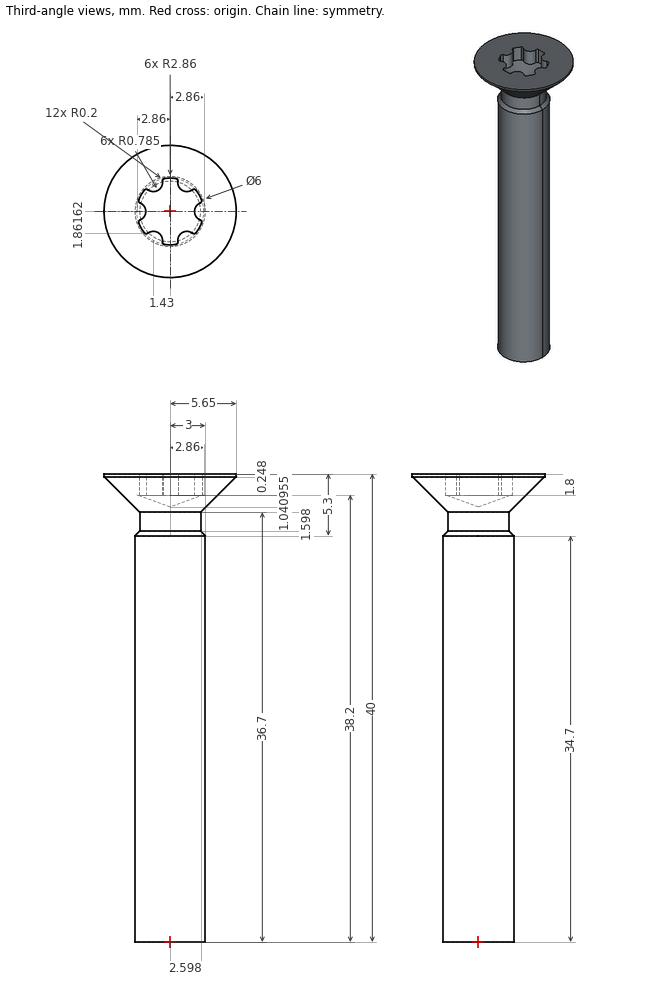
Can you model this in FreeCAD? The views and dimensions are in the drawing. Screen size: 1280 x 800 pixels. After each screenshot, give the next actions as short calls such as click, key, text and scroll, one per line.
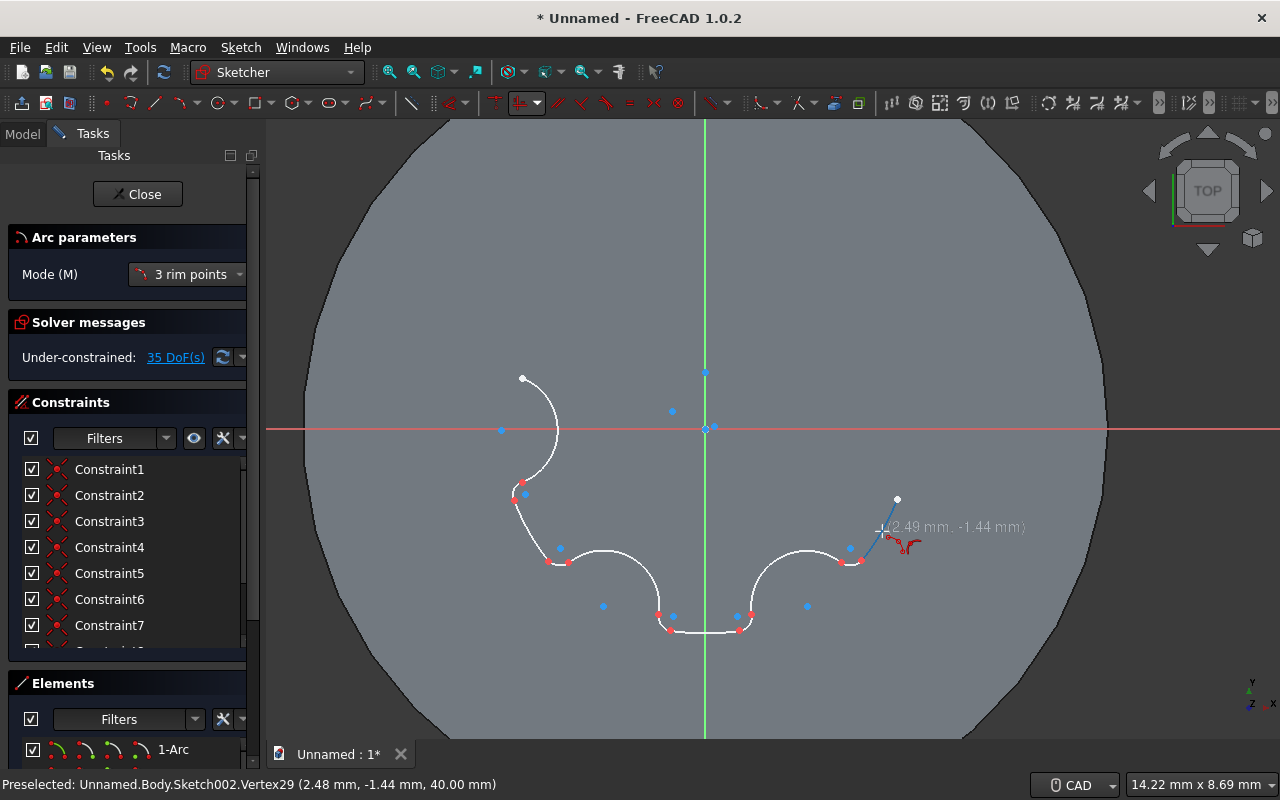
click(897, 500)
click(889, 481)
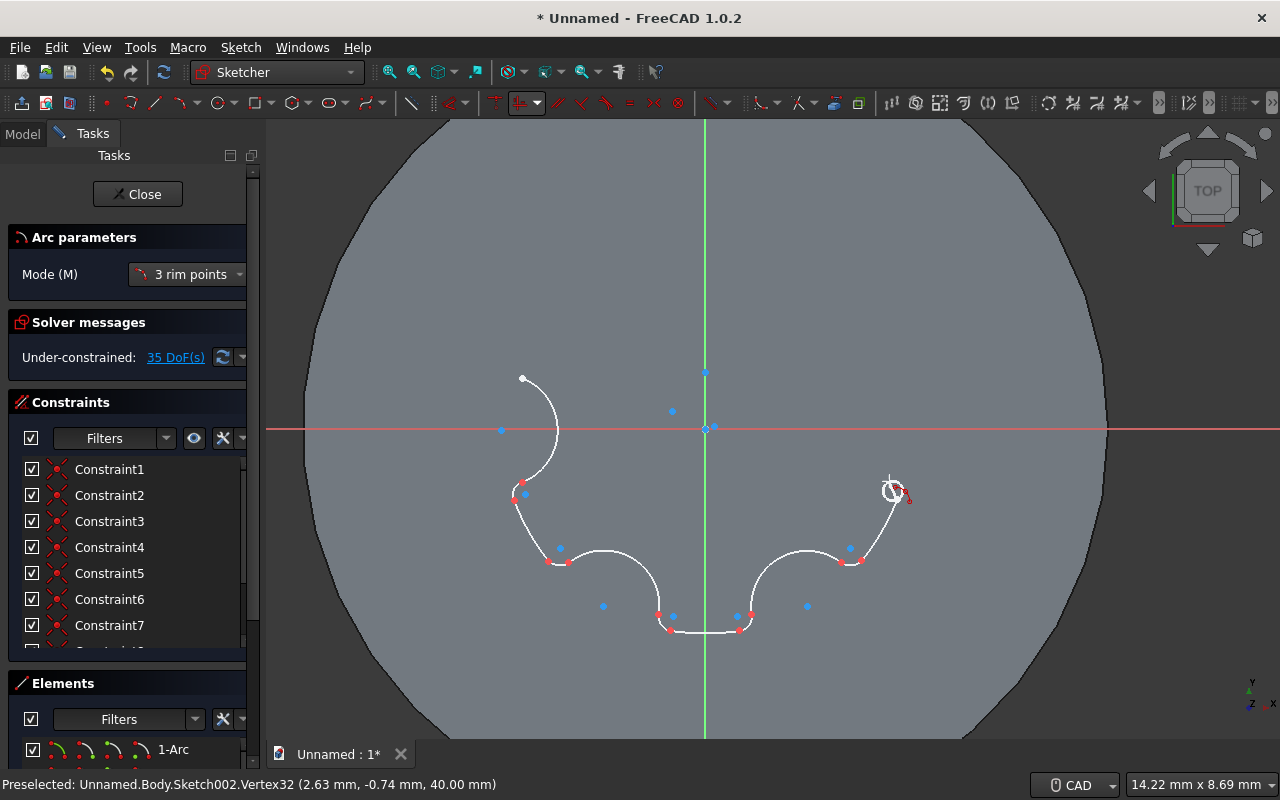
scroll(896, 489, up, 7)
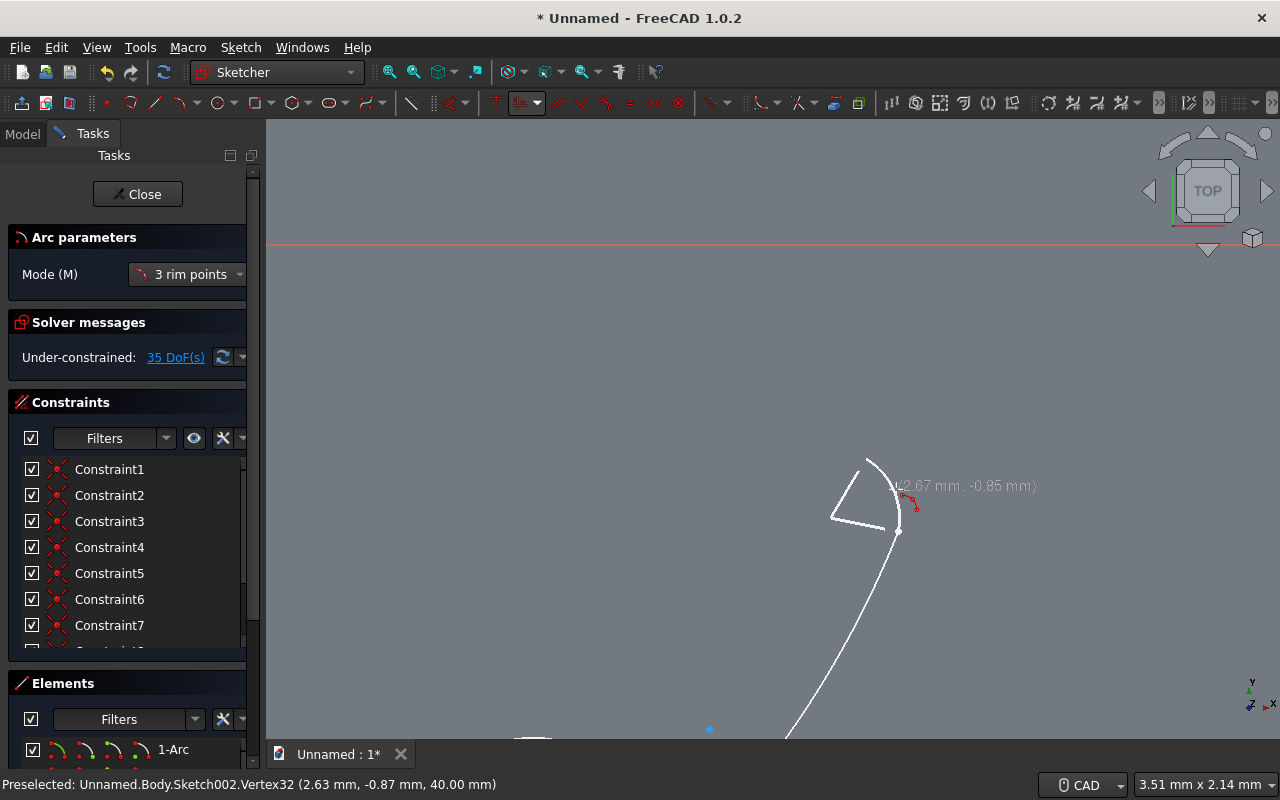
click(896, 486)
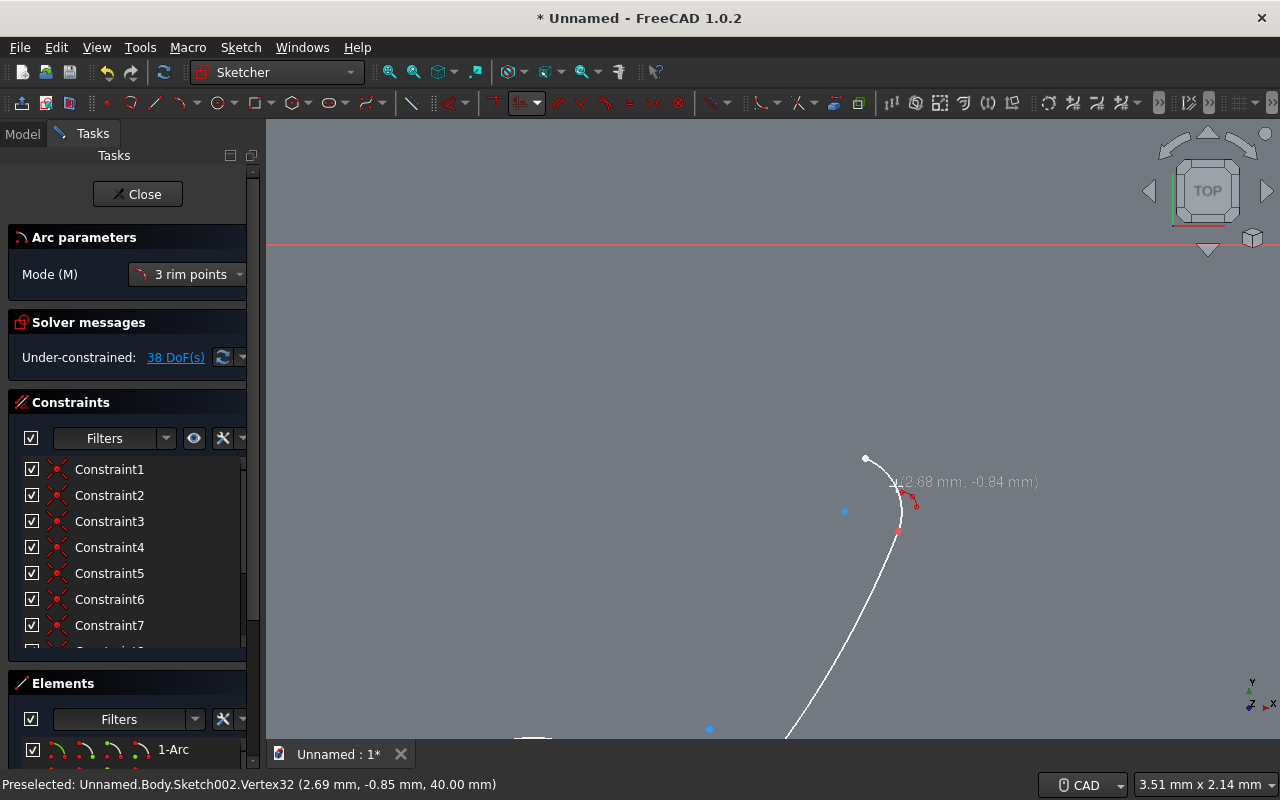
scroll(896, 489, down, 7)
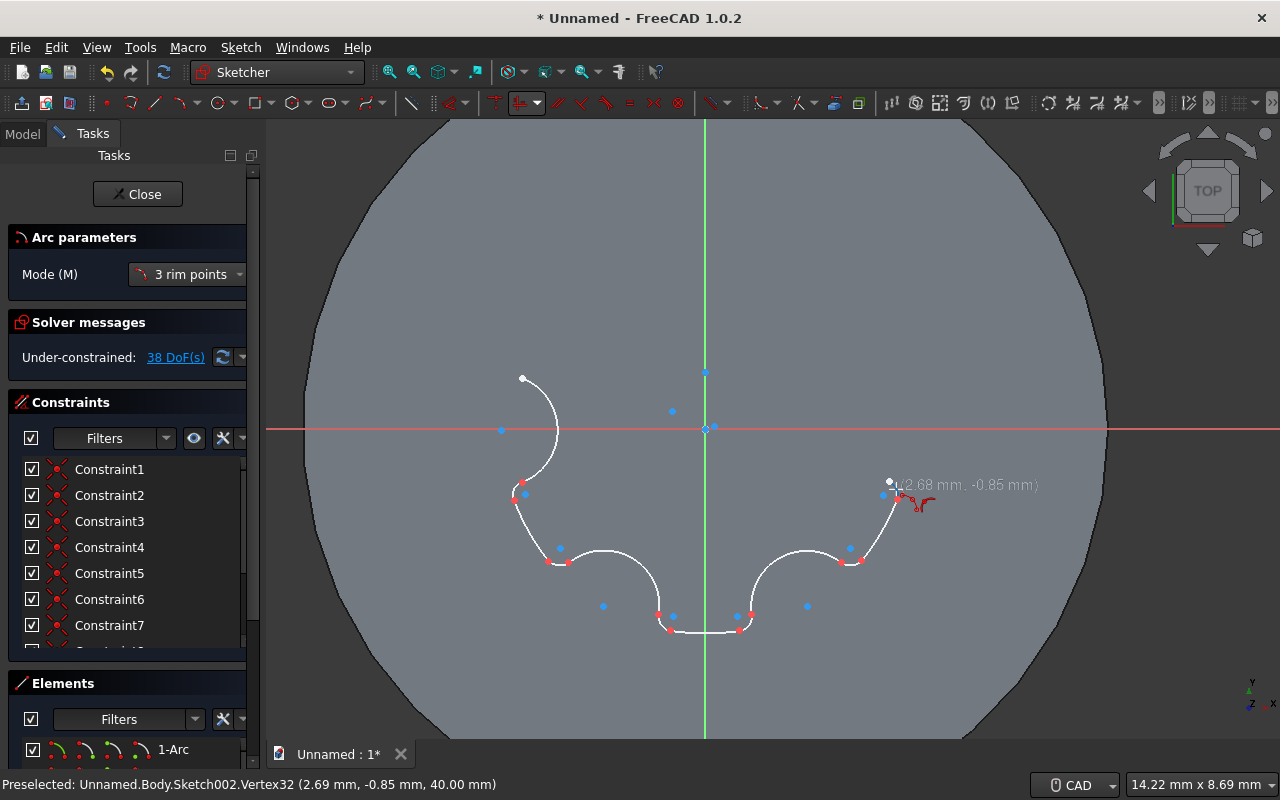
click(889, 482)
click(889, 377)
click(860, 404)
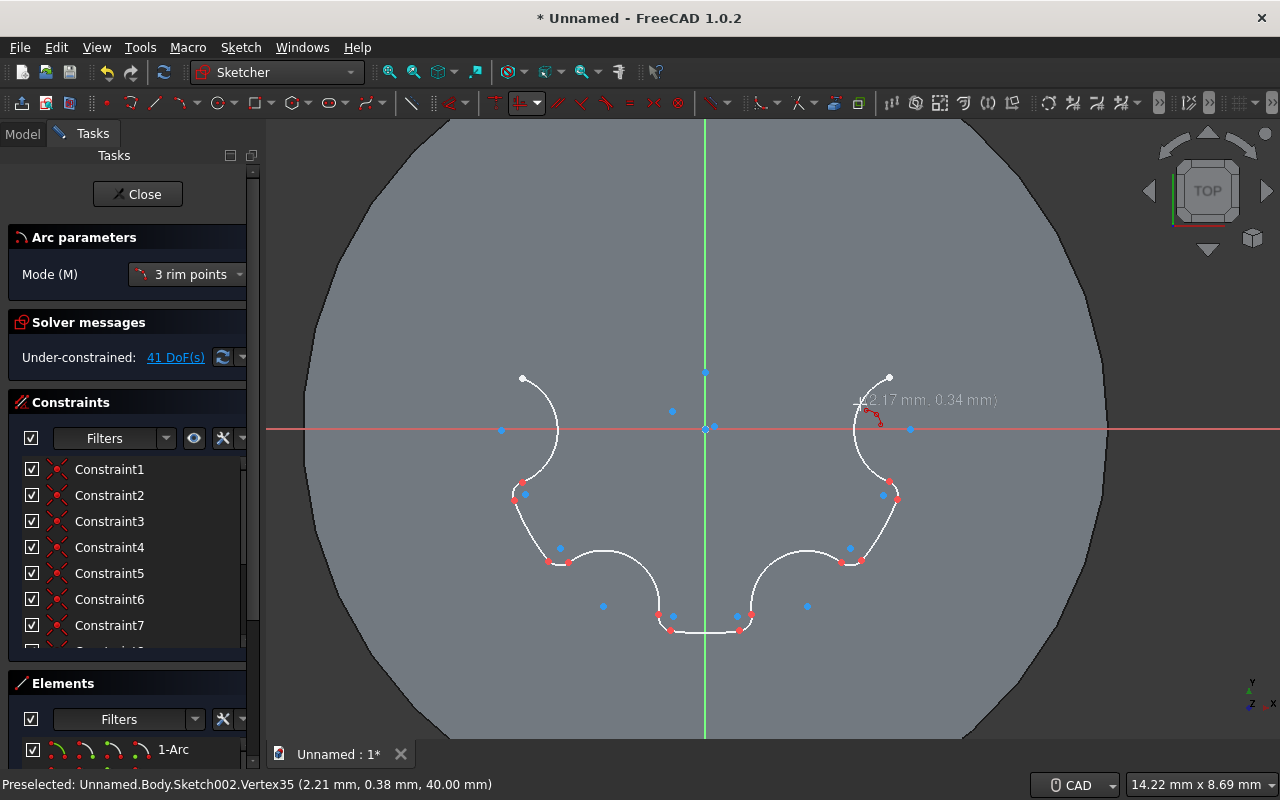
click(889, 378)
click(897, 359)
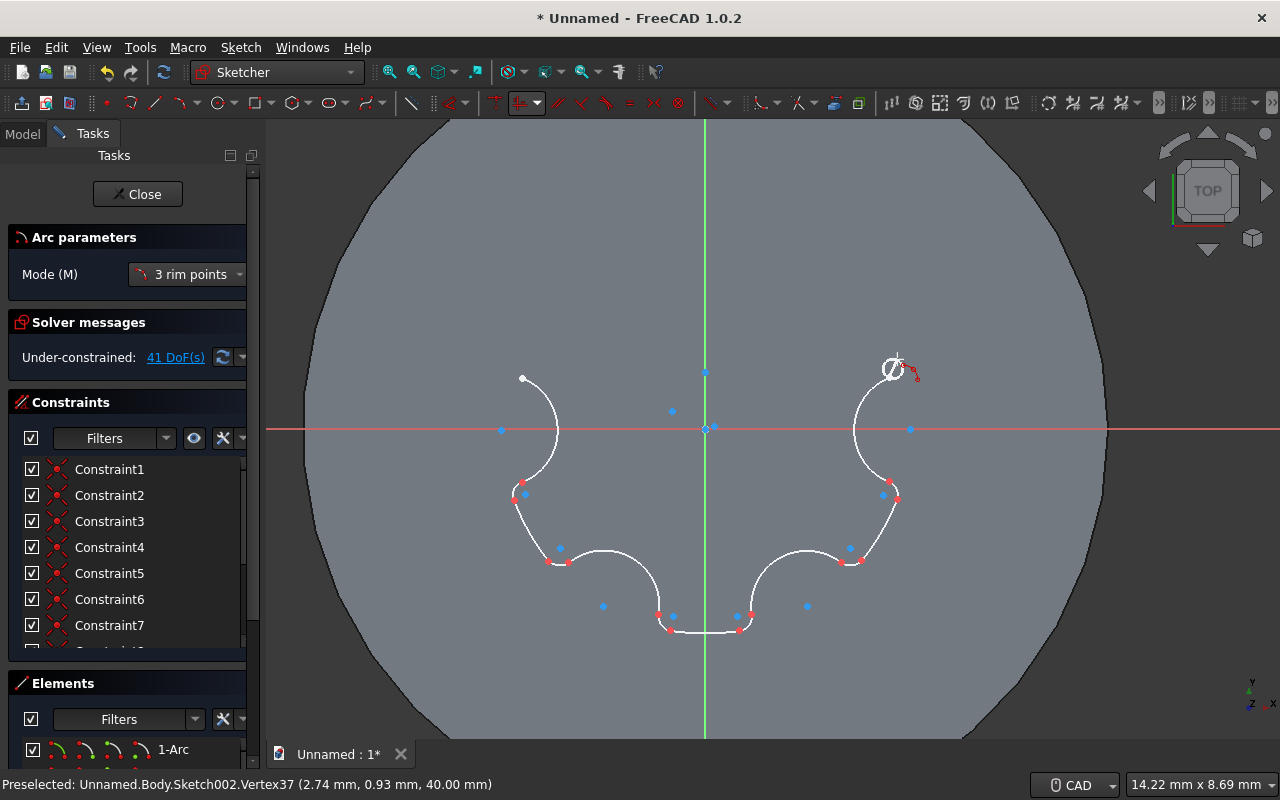
scroll(896, 370, up, 7)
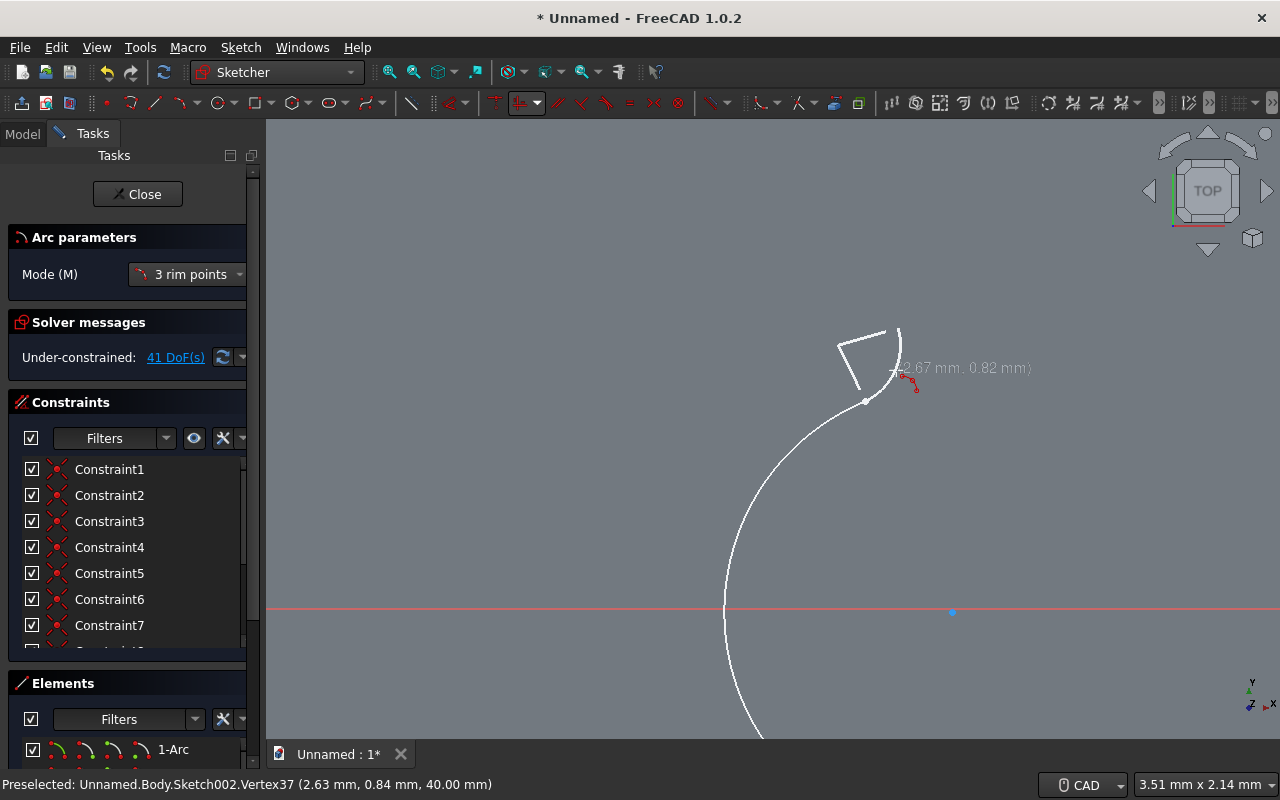
click(896, 368)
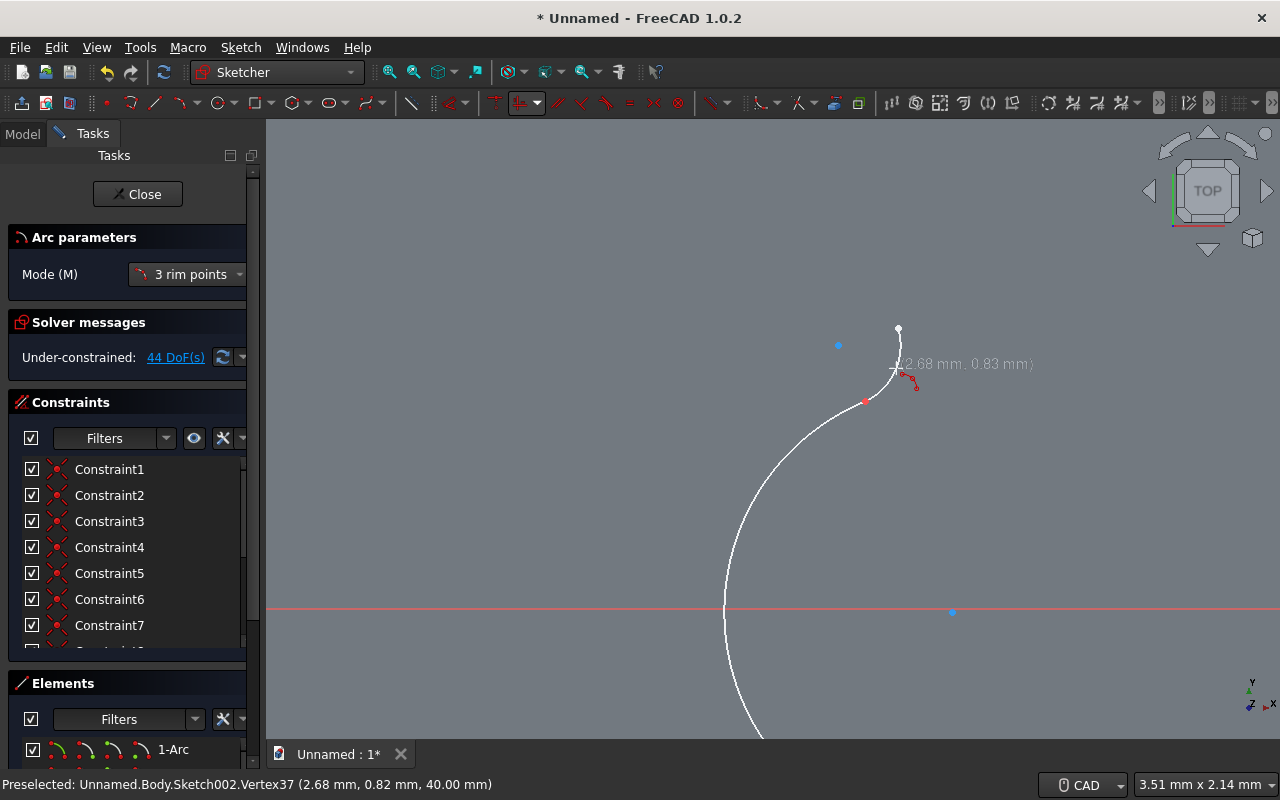
scroll(896, 370, down, 7)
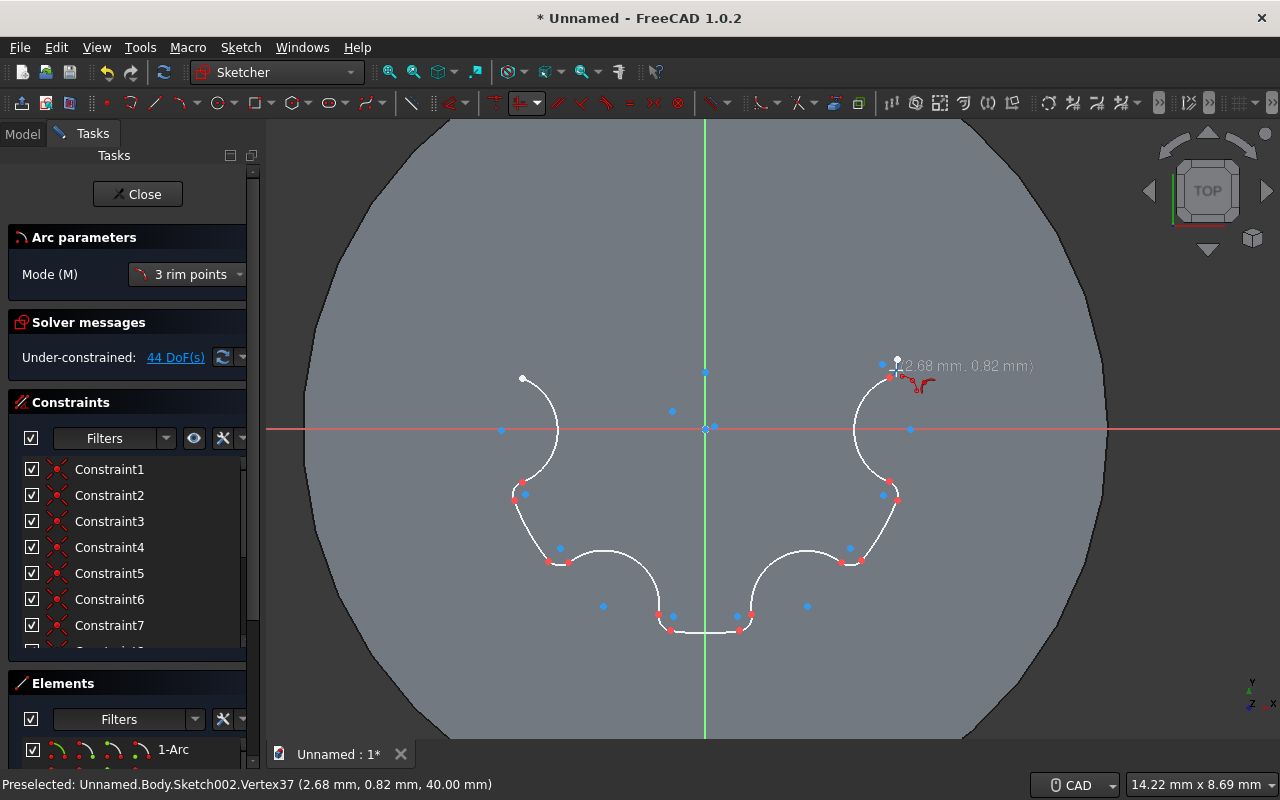
click(897, 360)
click(862, 299)